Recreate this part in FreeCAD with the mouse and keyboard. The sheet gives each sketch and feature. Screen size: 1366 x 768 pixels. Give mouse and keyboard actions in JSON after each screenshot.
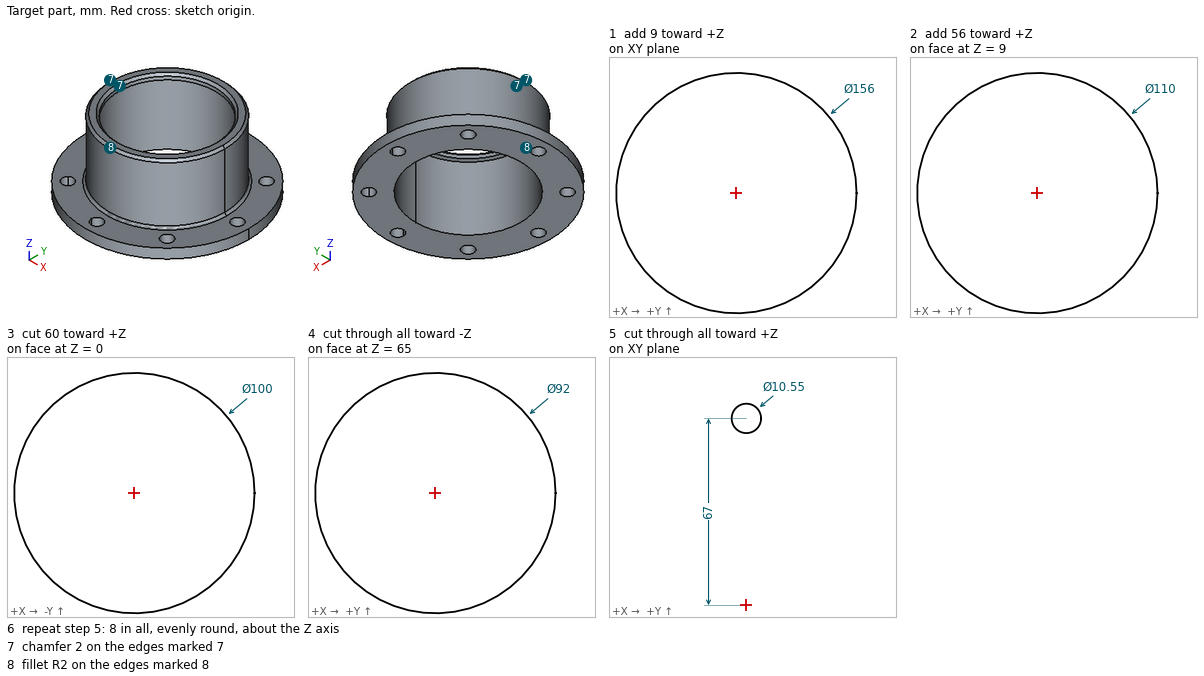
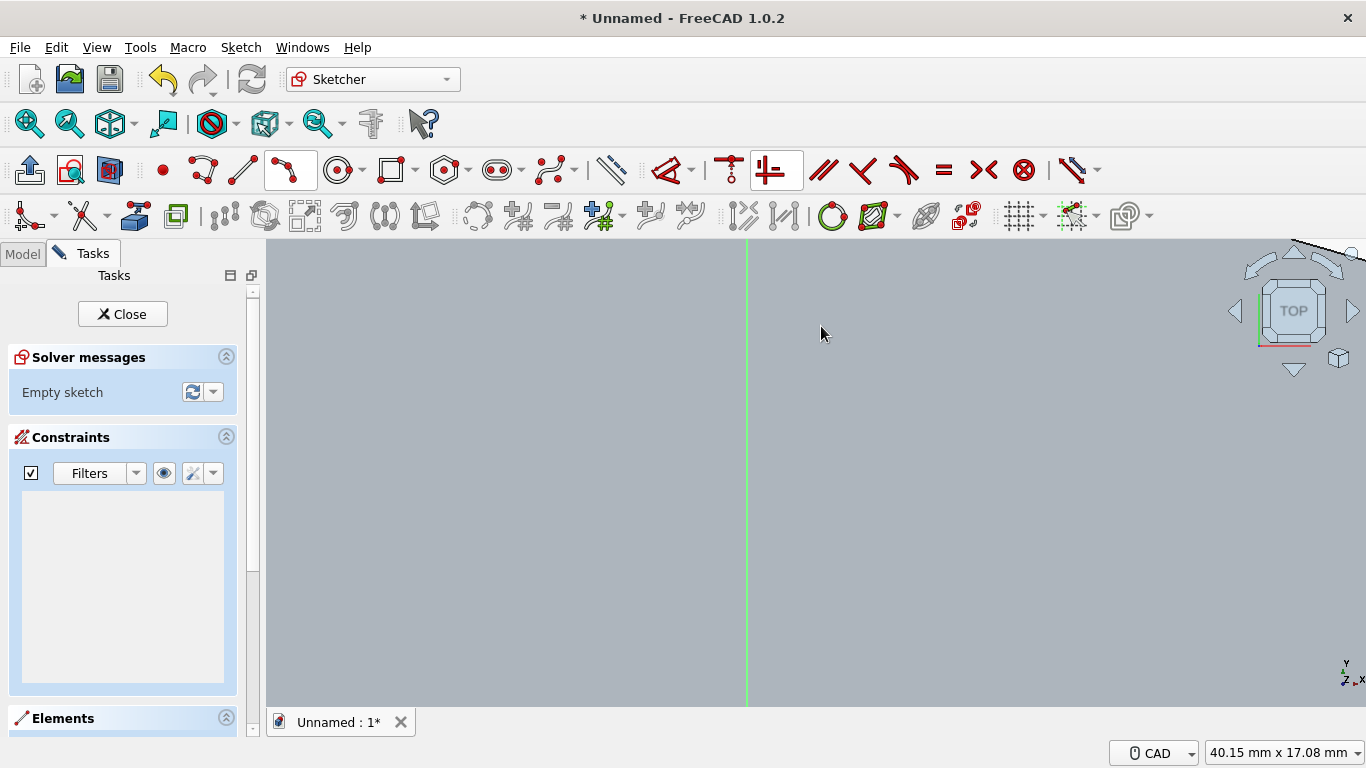
{"action": "left_click", "coordinate": [338, 170]}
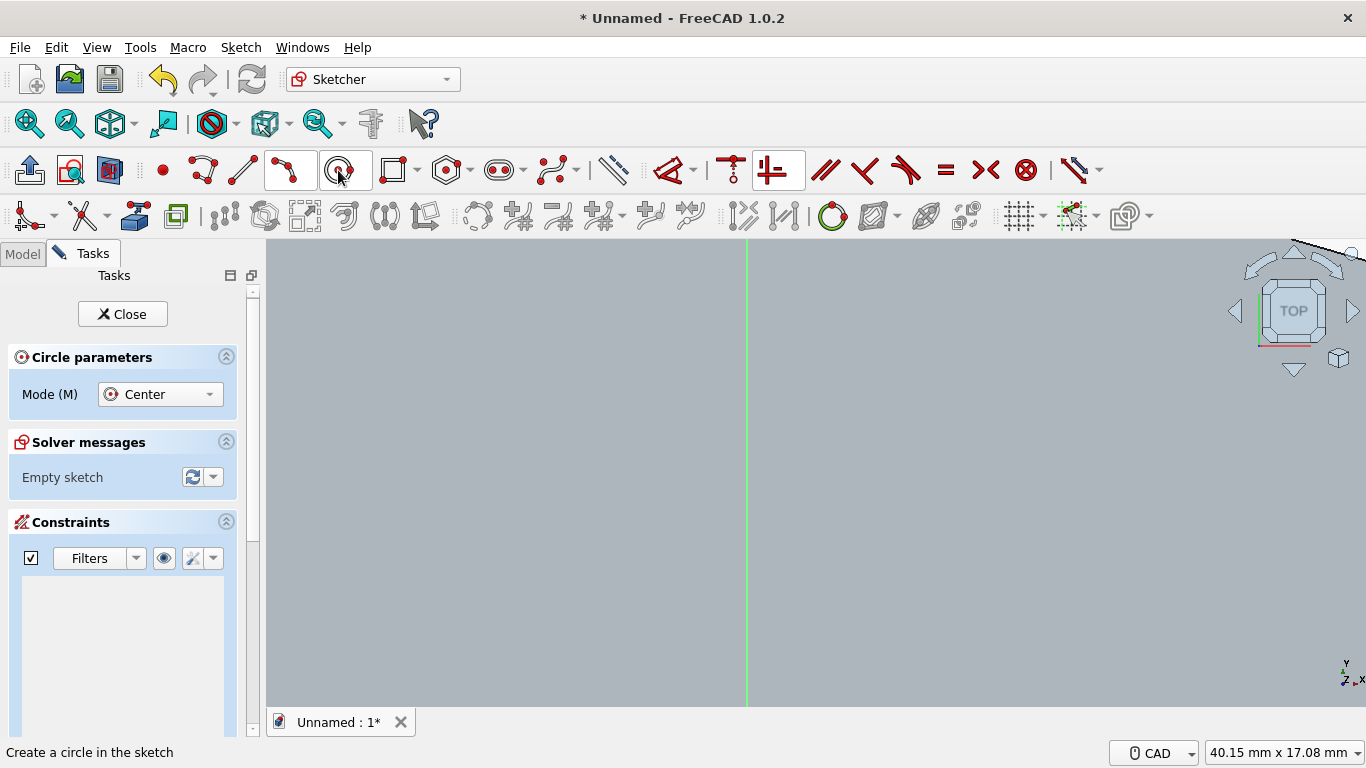
{"action": "left_click", "coordinate": [747, 467]}
{"action": "left_click", "coordinate": [850, 365]}
{"action": "key", "text": "Escape"}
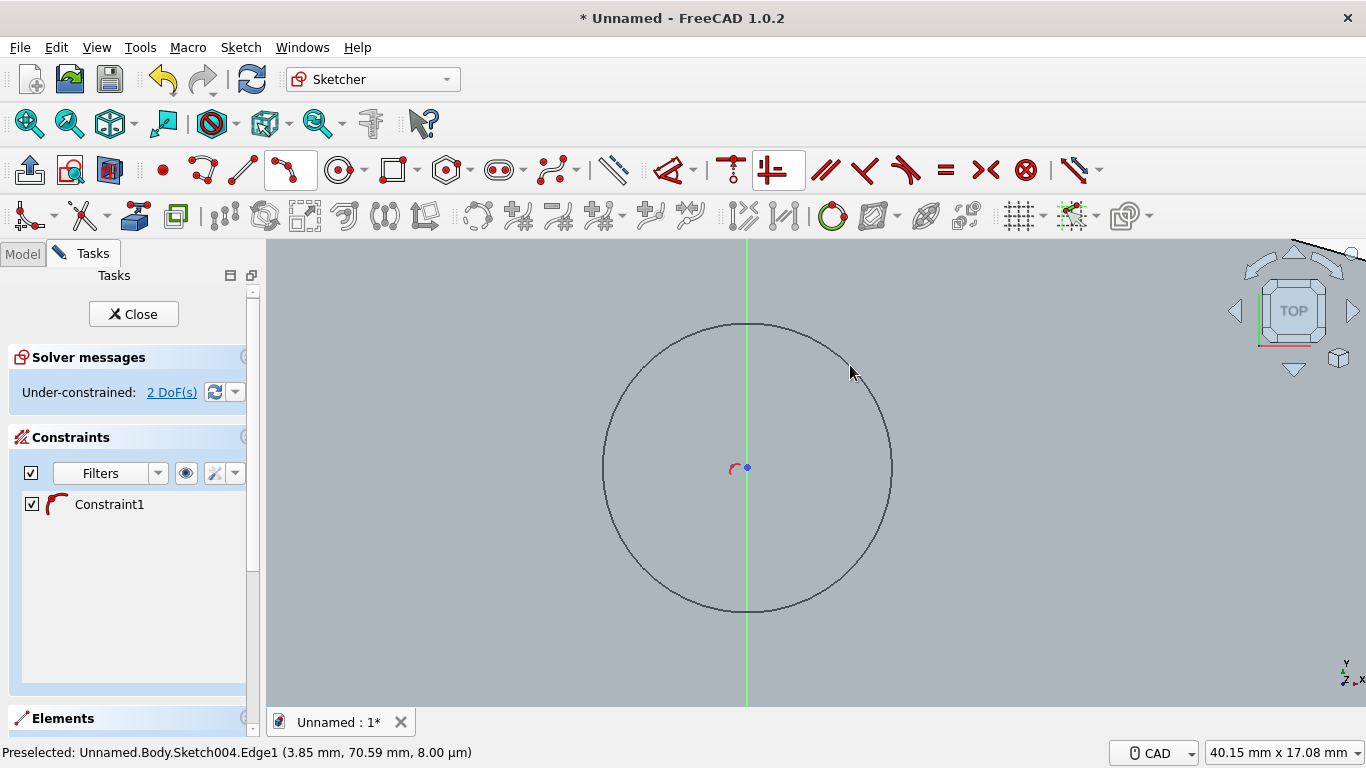
{"action": "key", "text": "d"}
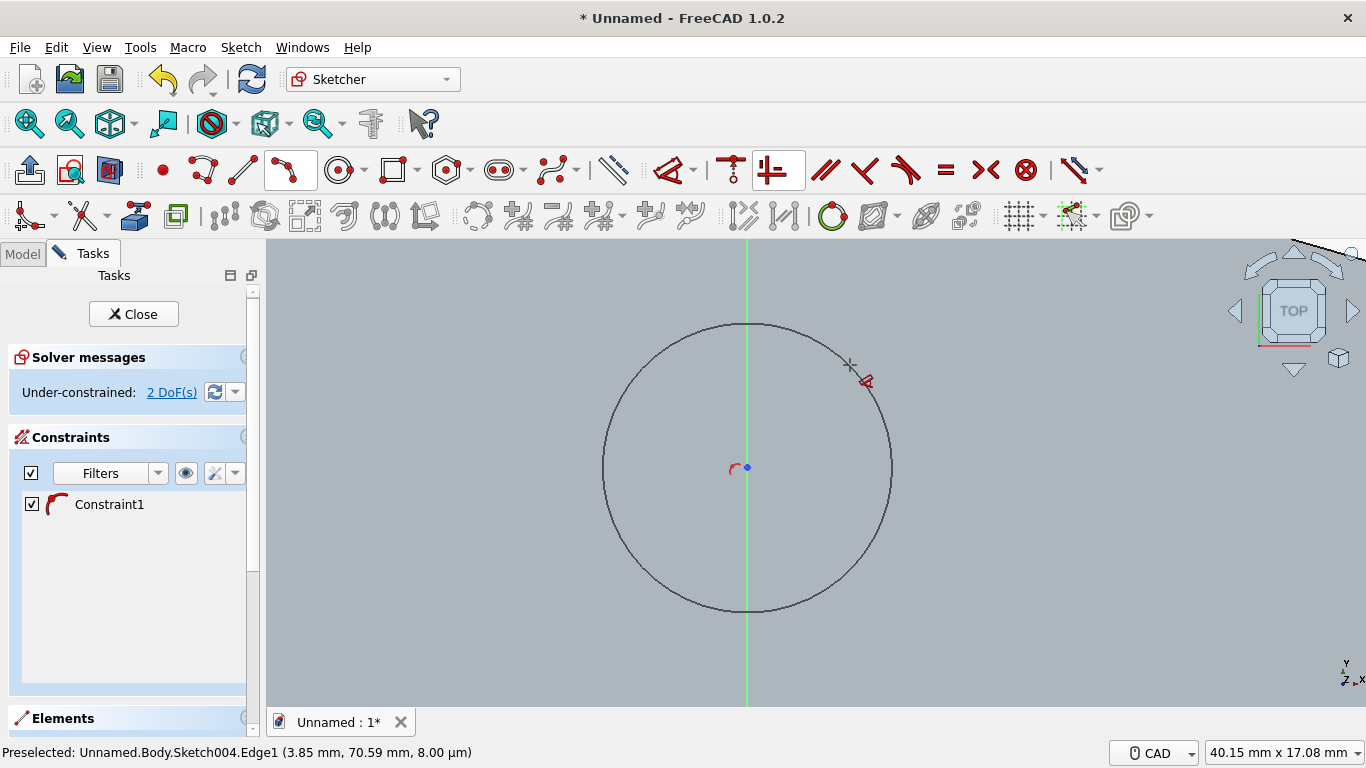
{"action": "left_click", "coordinate": [849, 365]}
{"action": "left_click", "coordinate": [871, 342]}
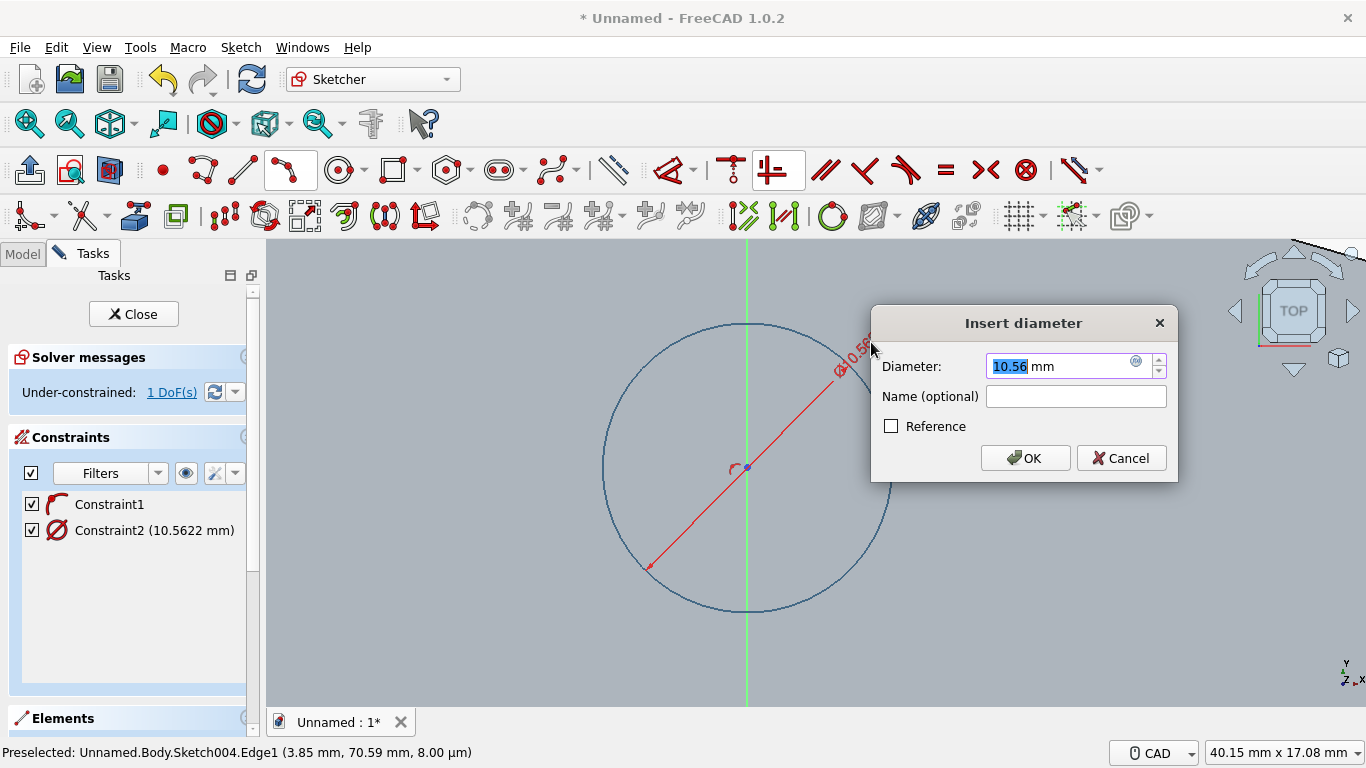
{"action": "type", "text": "10.55"}
{"action": "key", "text": "Return"}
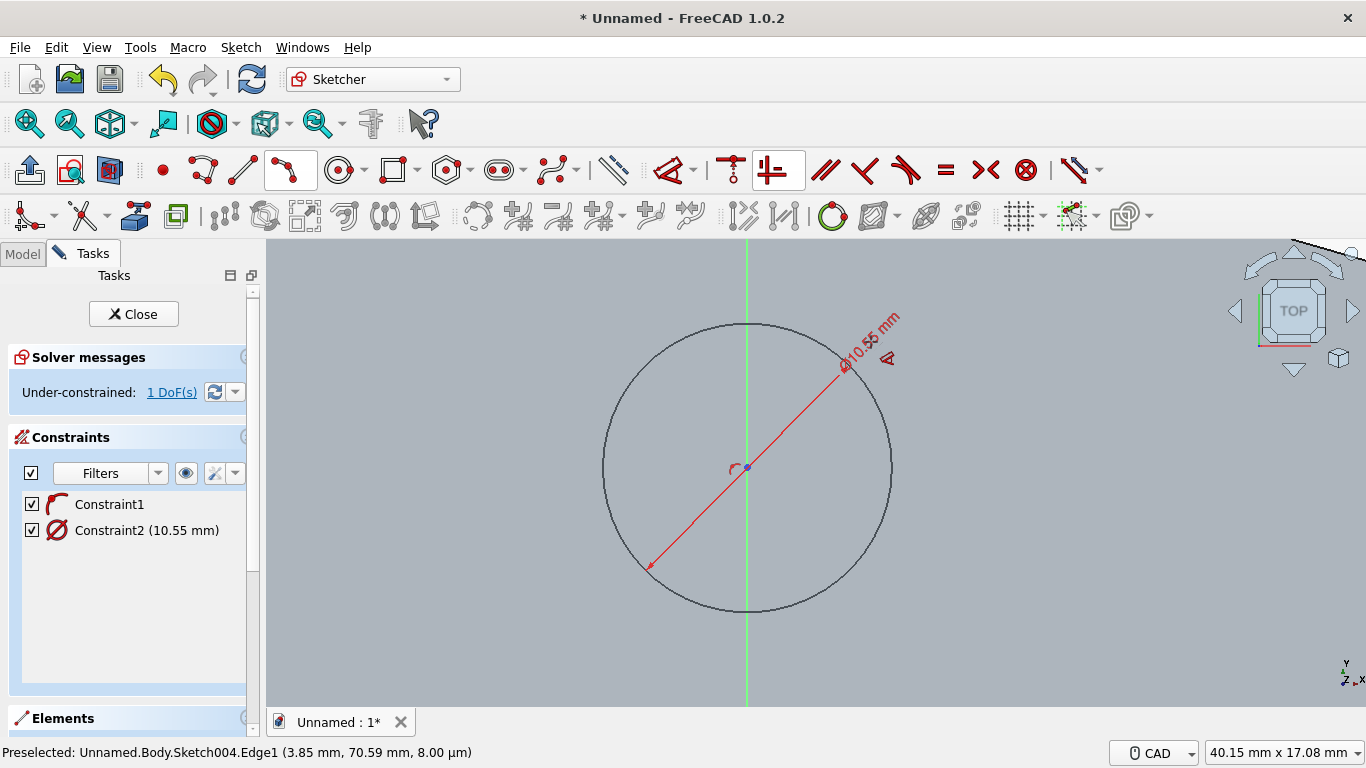
{"action": "left_click", "coordinate": [747, 468]}
{"action": "left_click", "coordinate": [781, 574]}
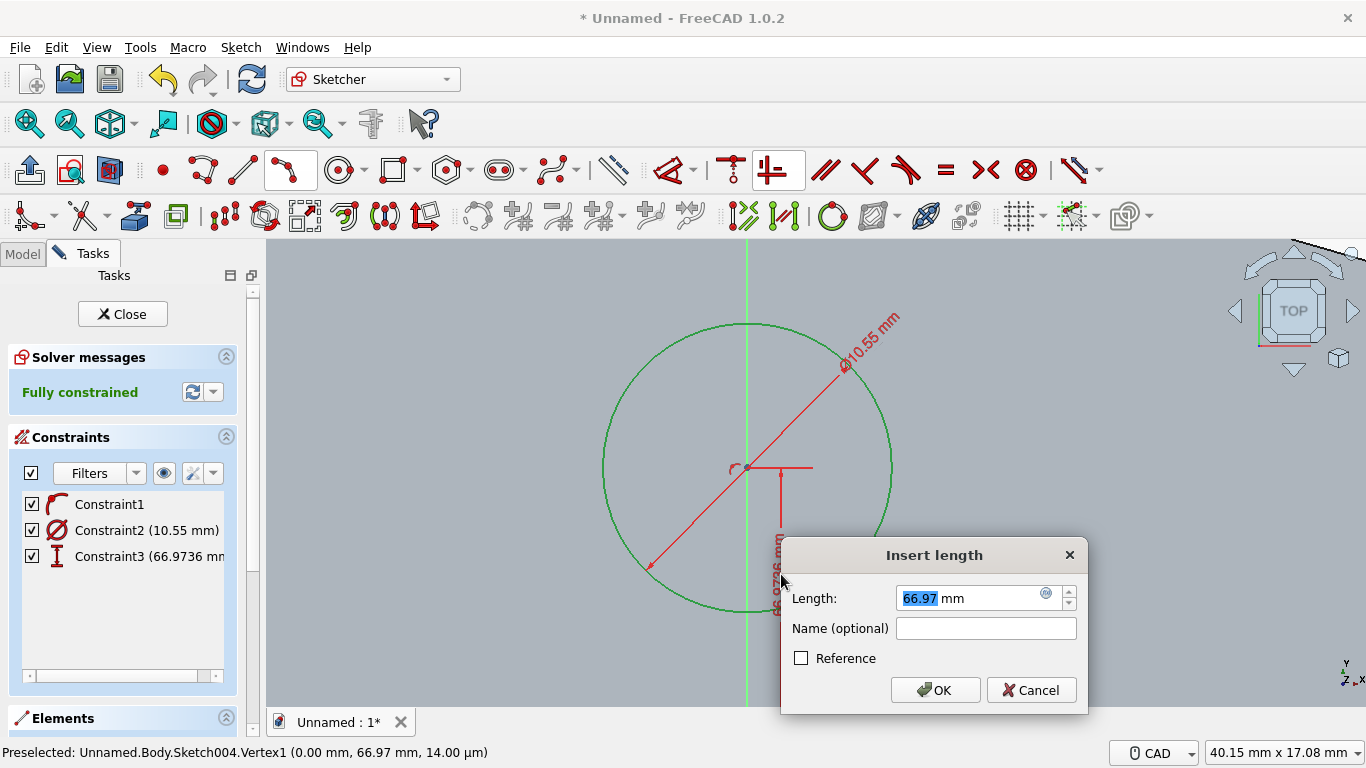
{"action": "type", "text": "67"}
{"action": "key", "text": "Return"}
{"action": "key", "text": "Escape"}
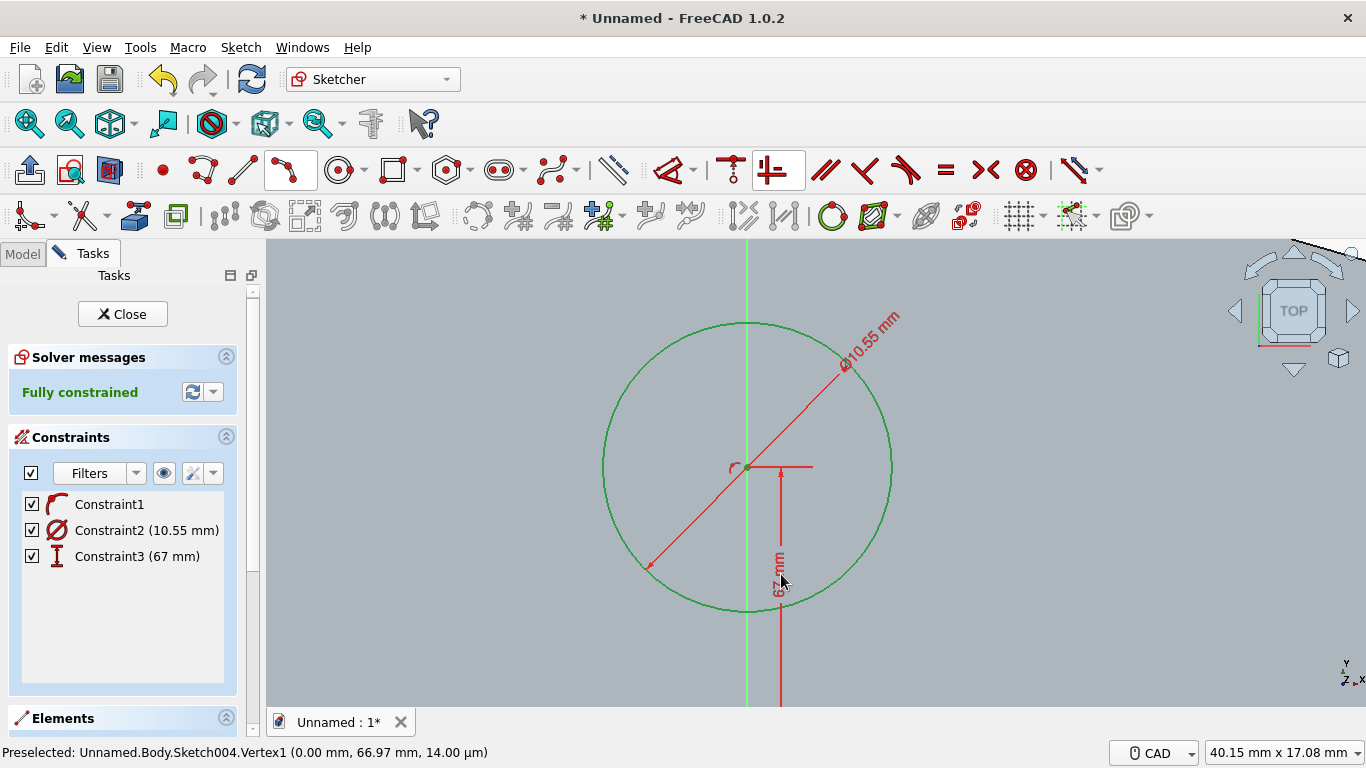
{"action": "left_click", "coordinate": [123, 314]}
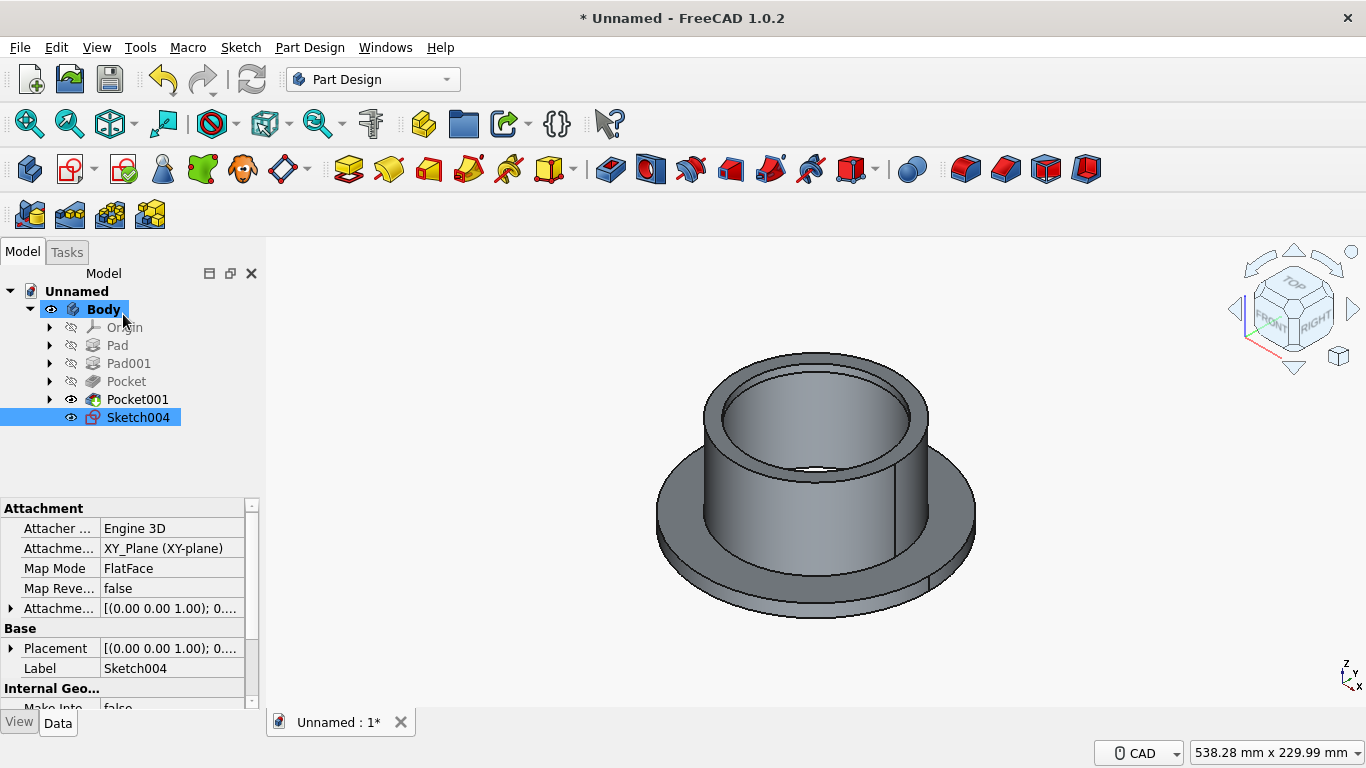
{"action": "left_click", "coordinate": [612, 170]}